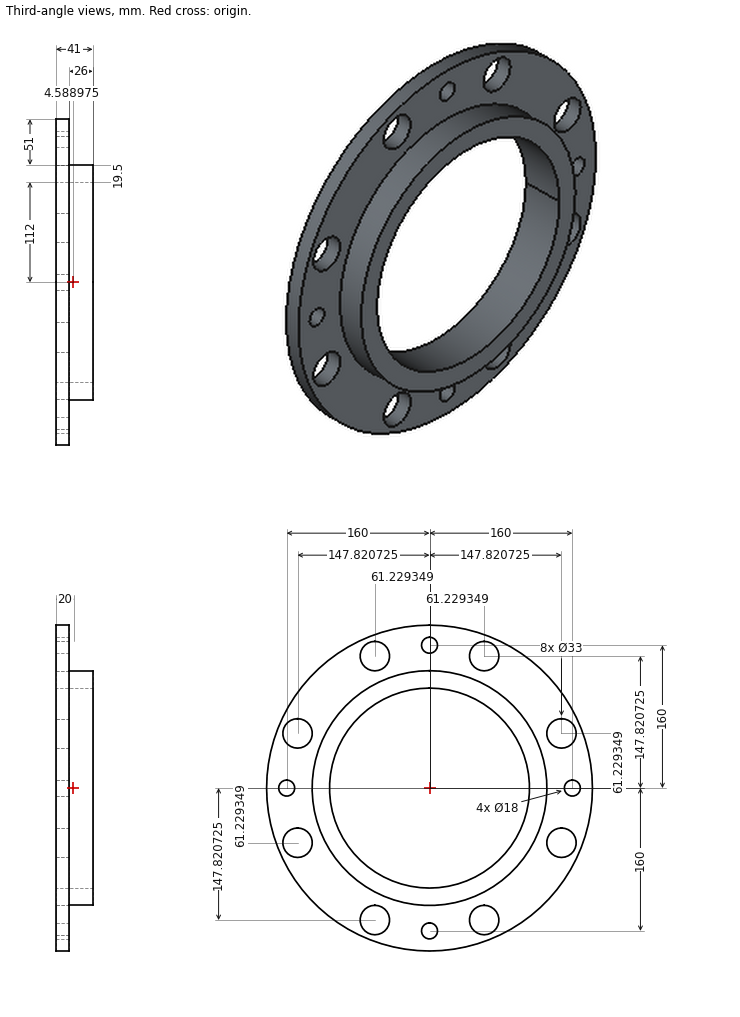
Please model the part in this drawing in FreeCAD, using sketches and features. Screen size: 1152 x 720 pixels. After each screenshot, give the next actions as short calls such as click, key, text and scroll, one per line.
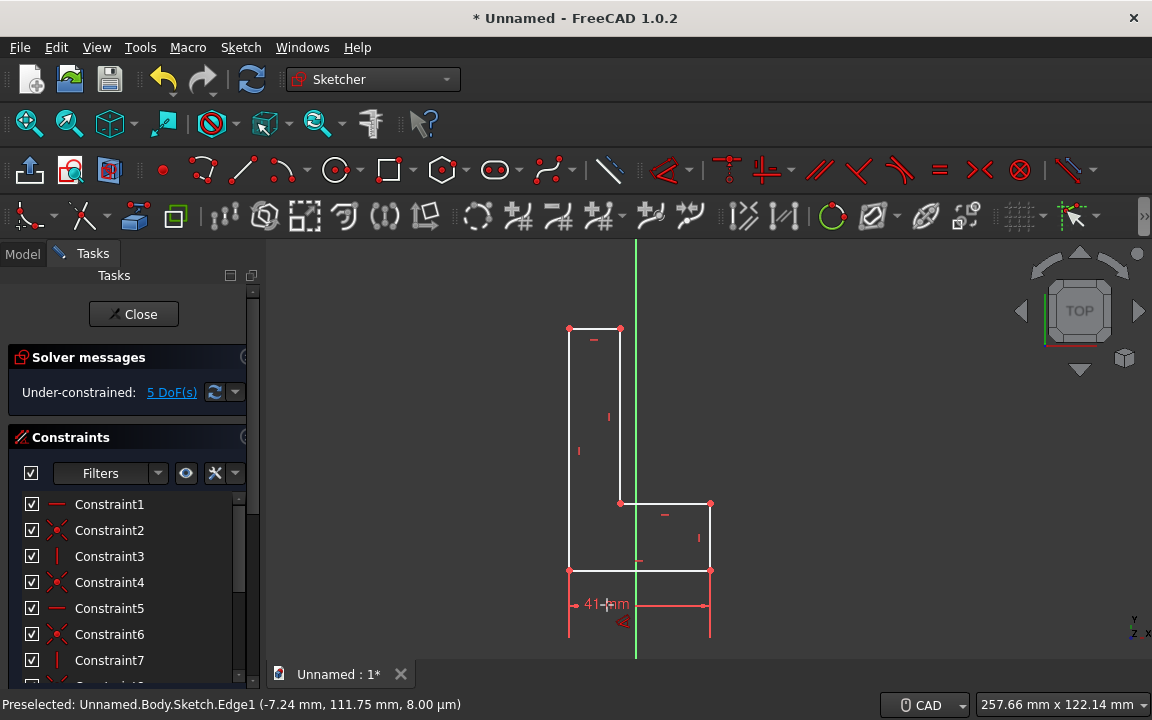
click(683, 504)
click(665, 538)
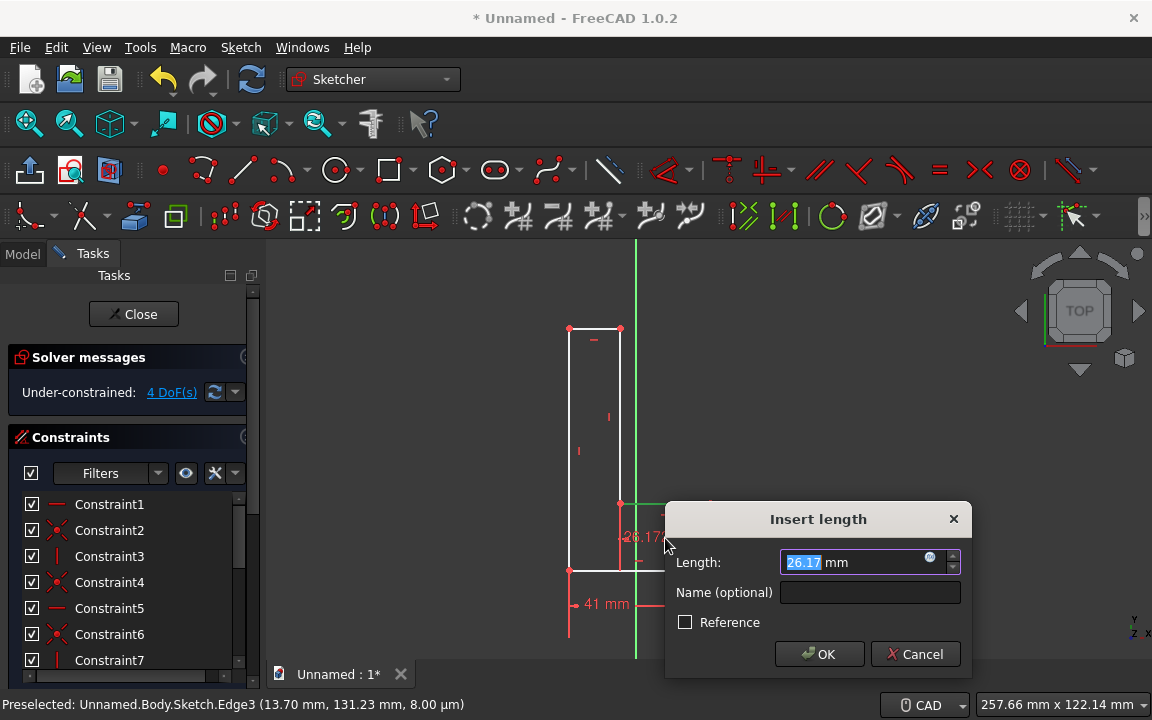
text(26)
key(Return)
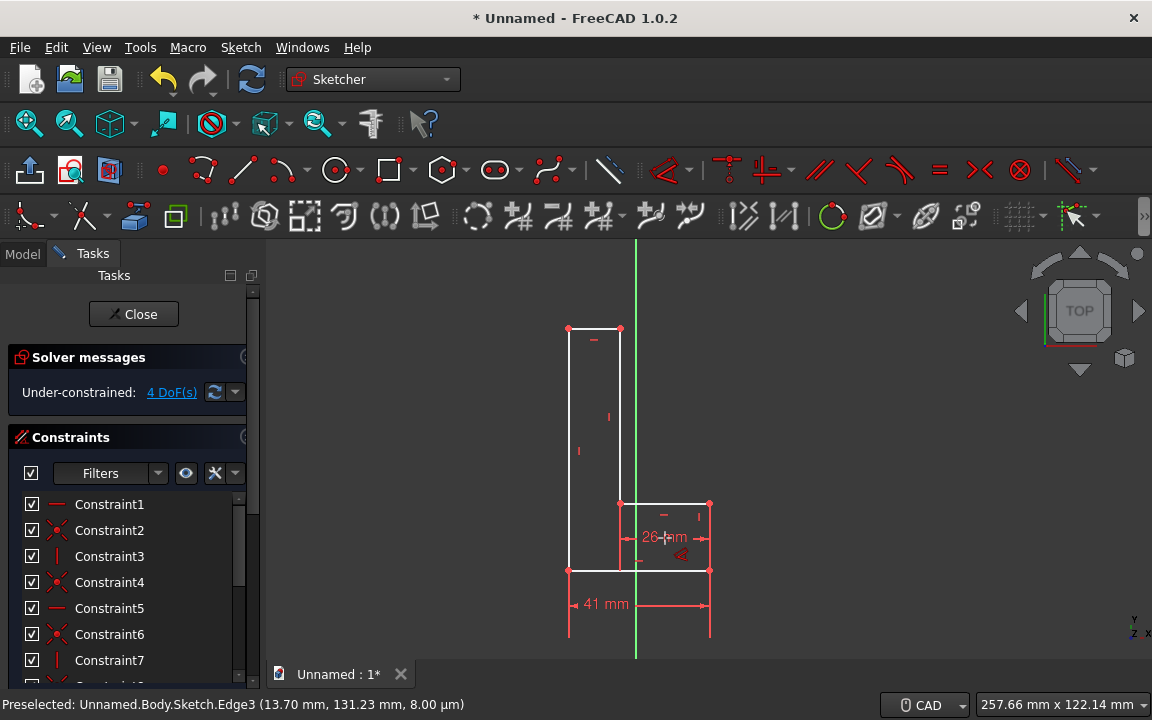
click(620, 452)
click(586, 417)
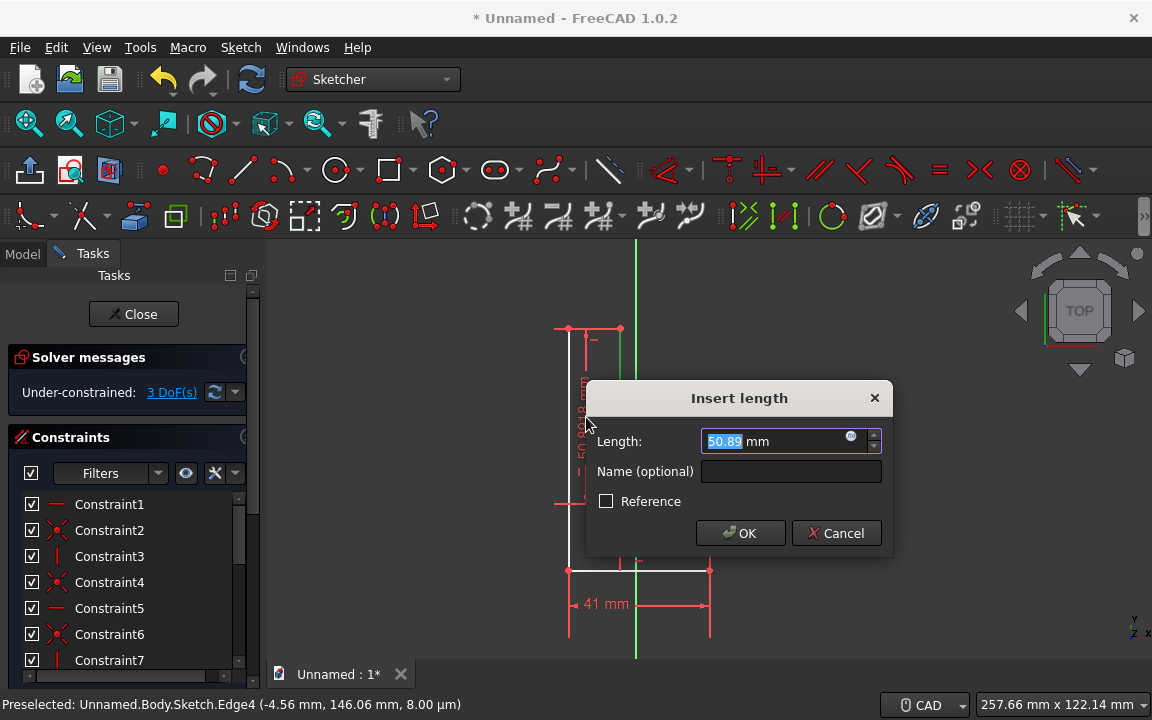
text(51)
key(Return)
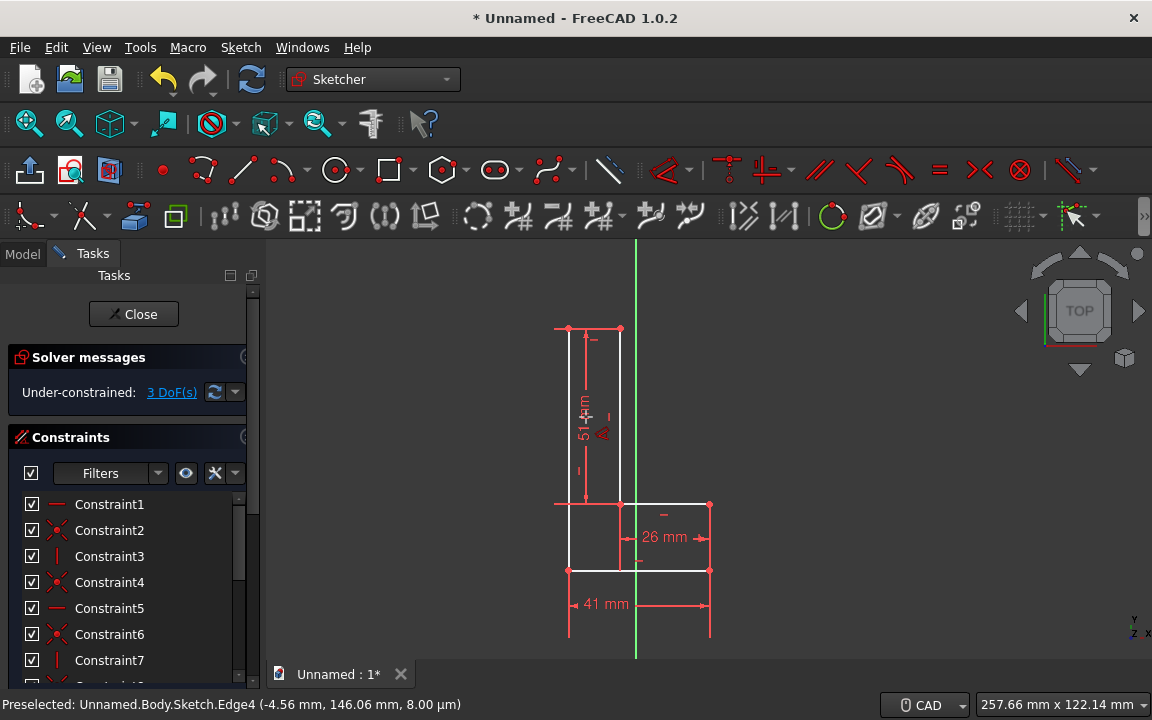
click(710, 551)
click(744, 538)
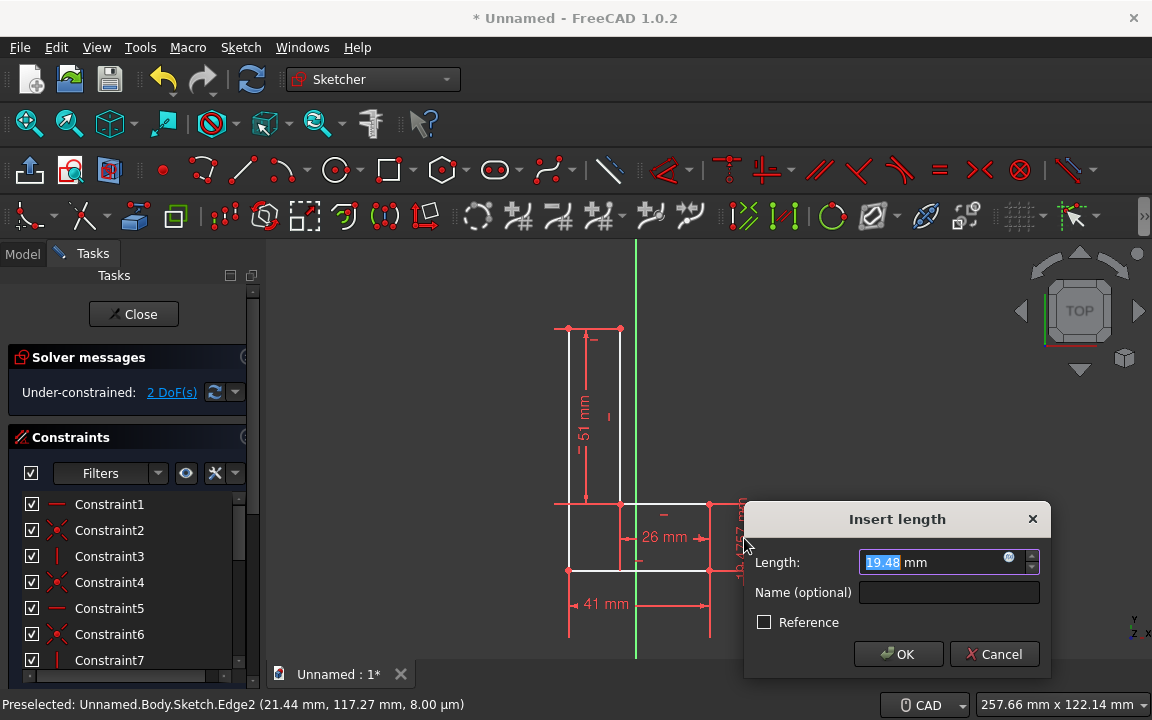
text(19.5)
key(Return)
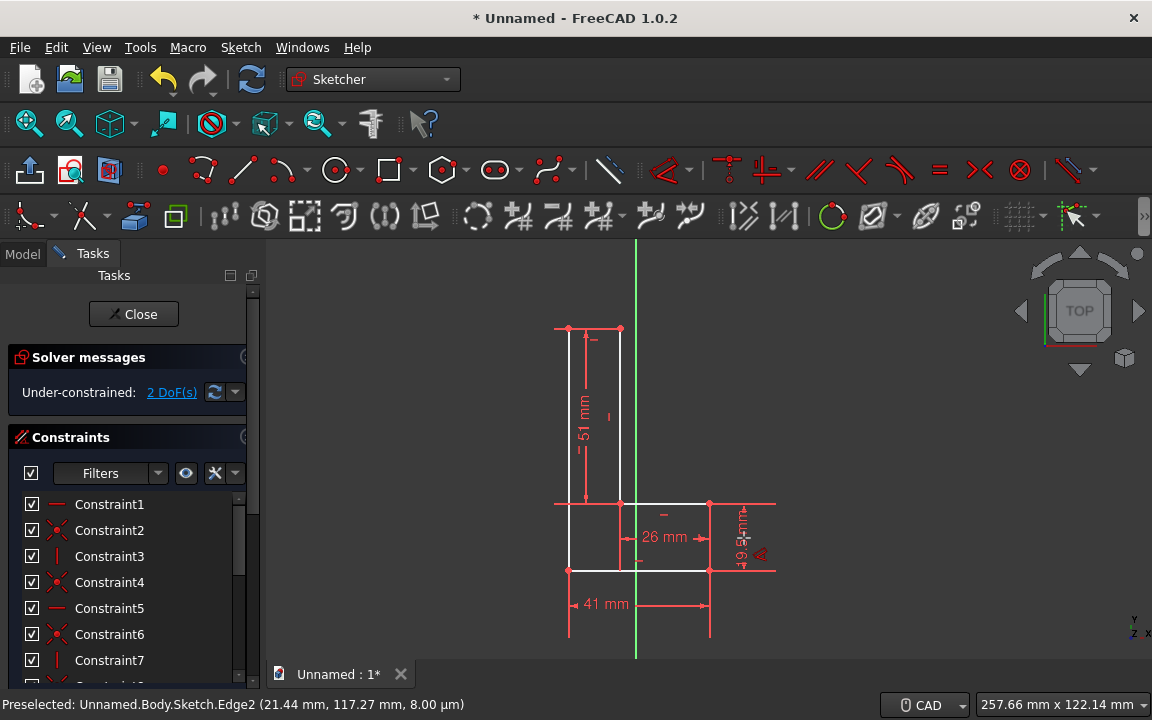
click(569, 571)
click(535, 601)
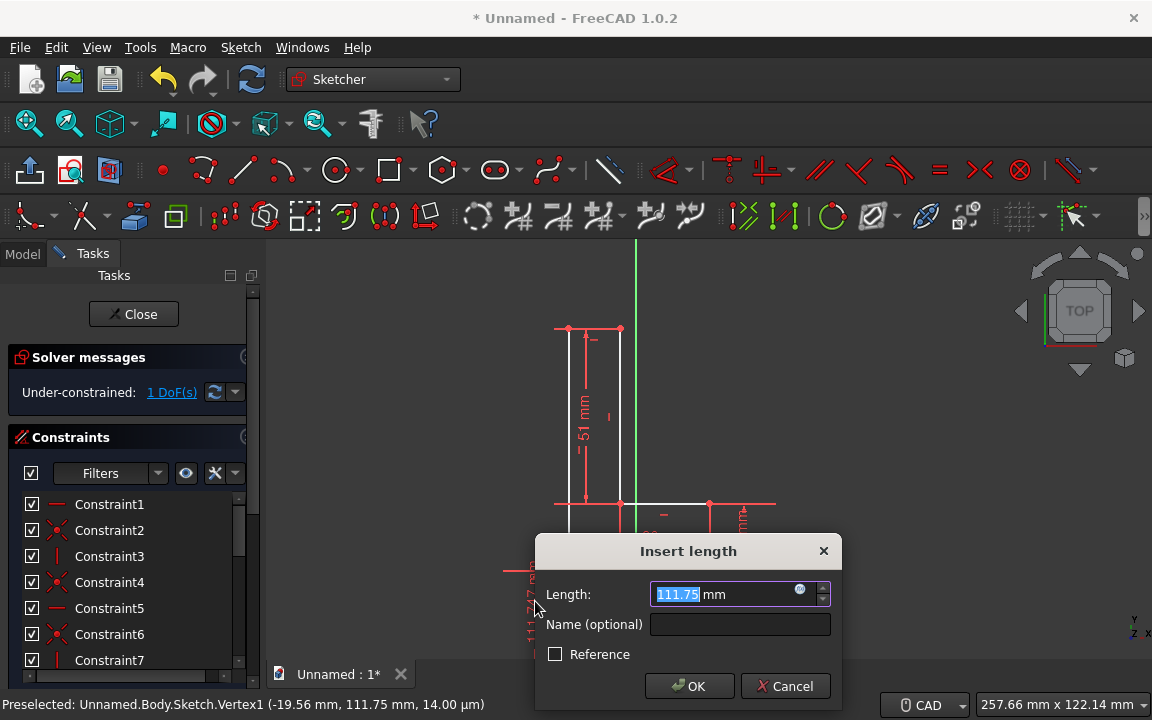
text(112)
key(Return)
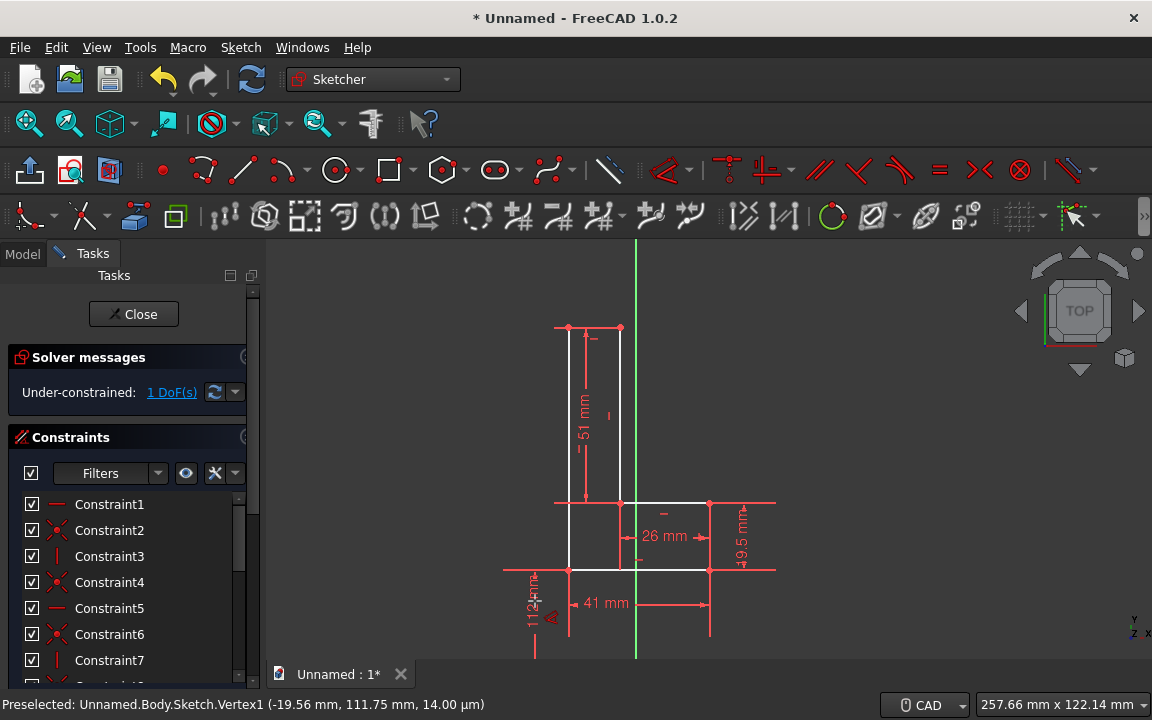
scroll(620, 503, up, 5)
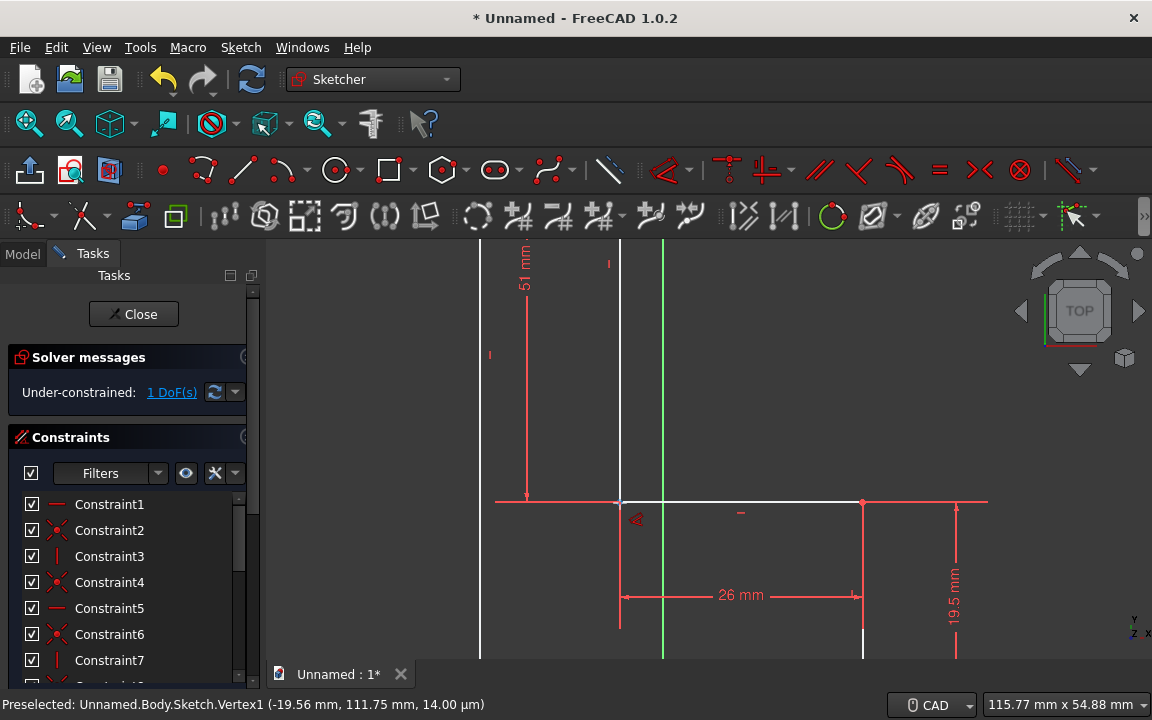
click(620, 502)
click(641, 468)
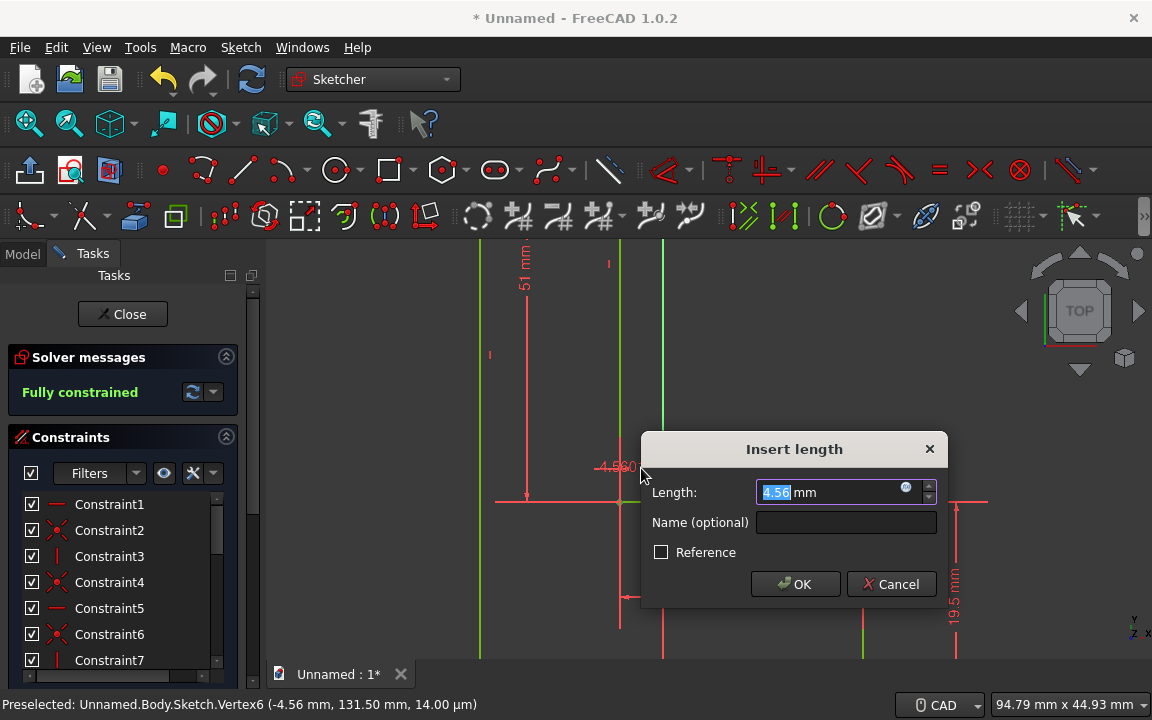
text(4.588975)
key(Return)
key(Escape)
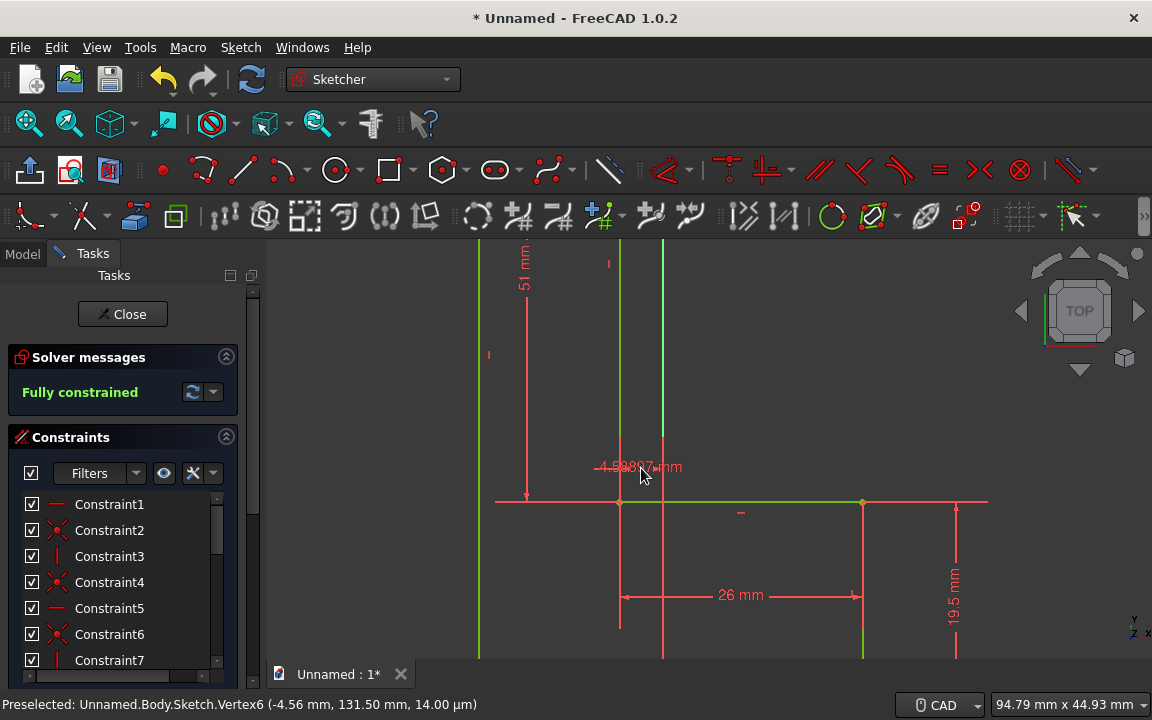
click(123, 314)